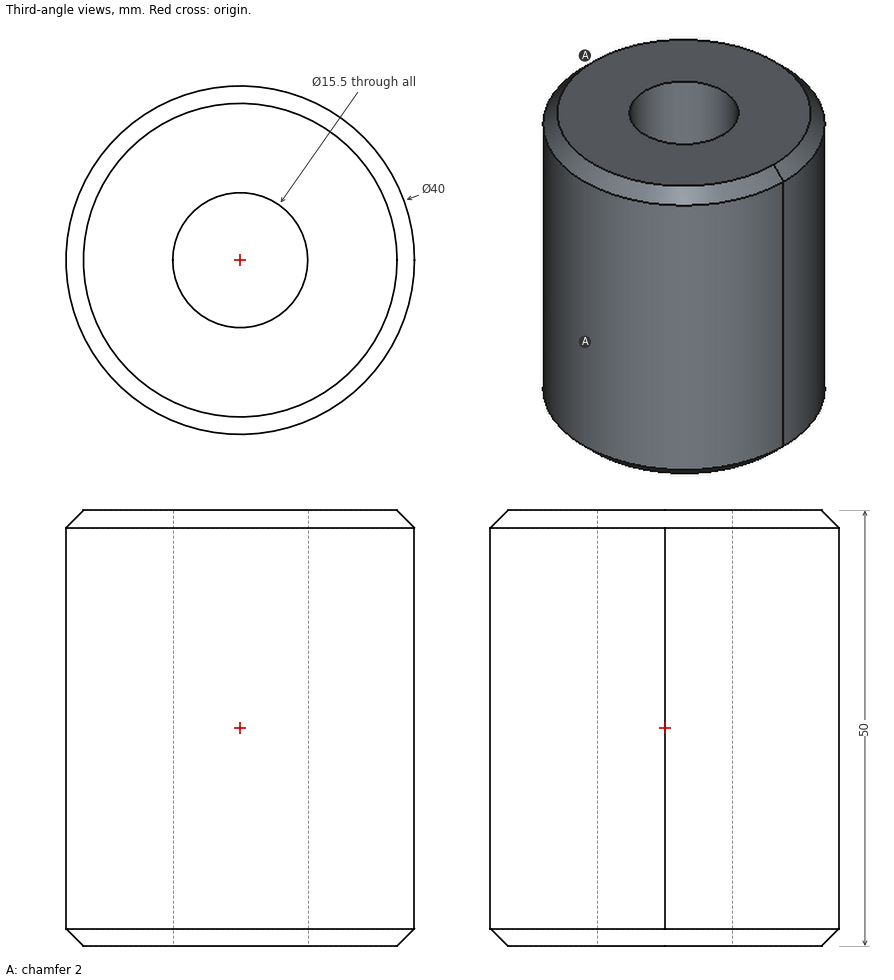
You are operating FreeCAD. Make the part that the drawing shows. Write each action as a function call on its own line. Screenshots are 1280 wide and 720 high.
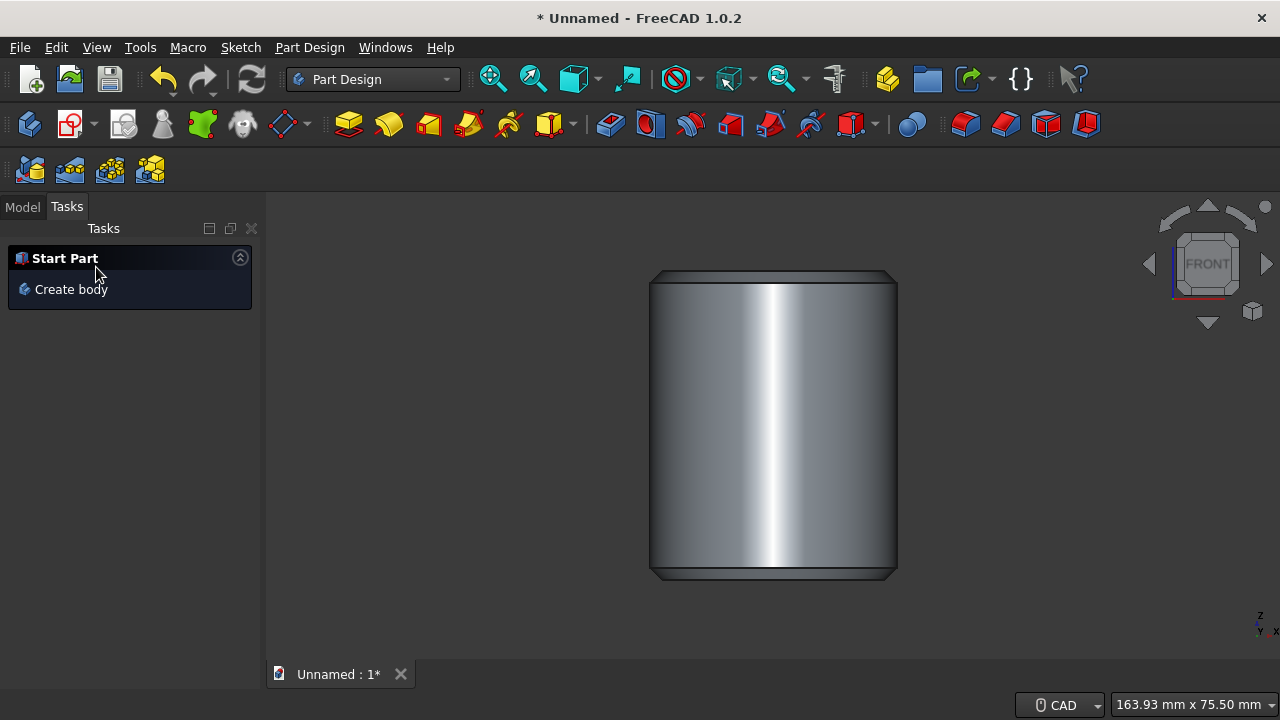
key(0)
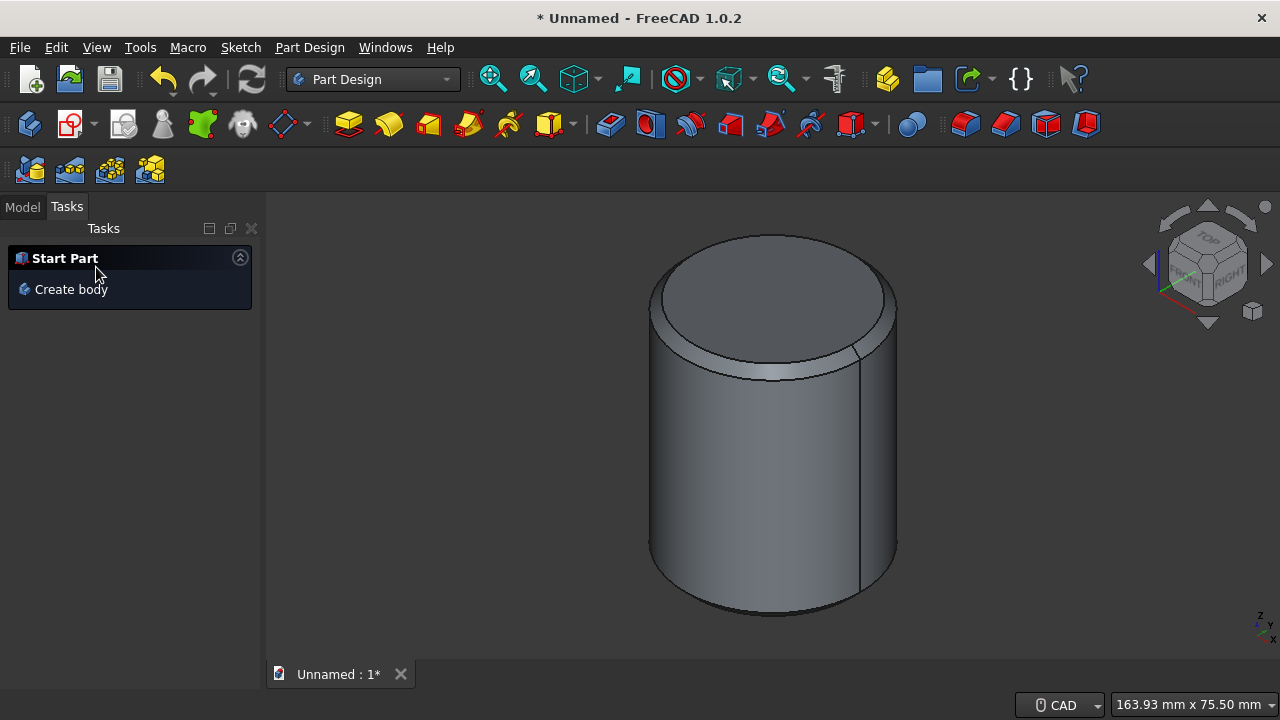
click(773, 298)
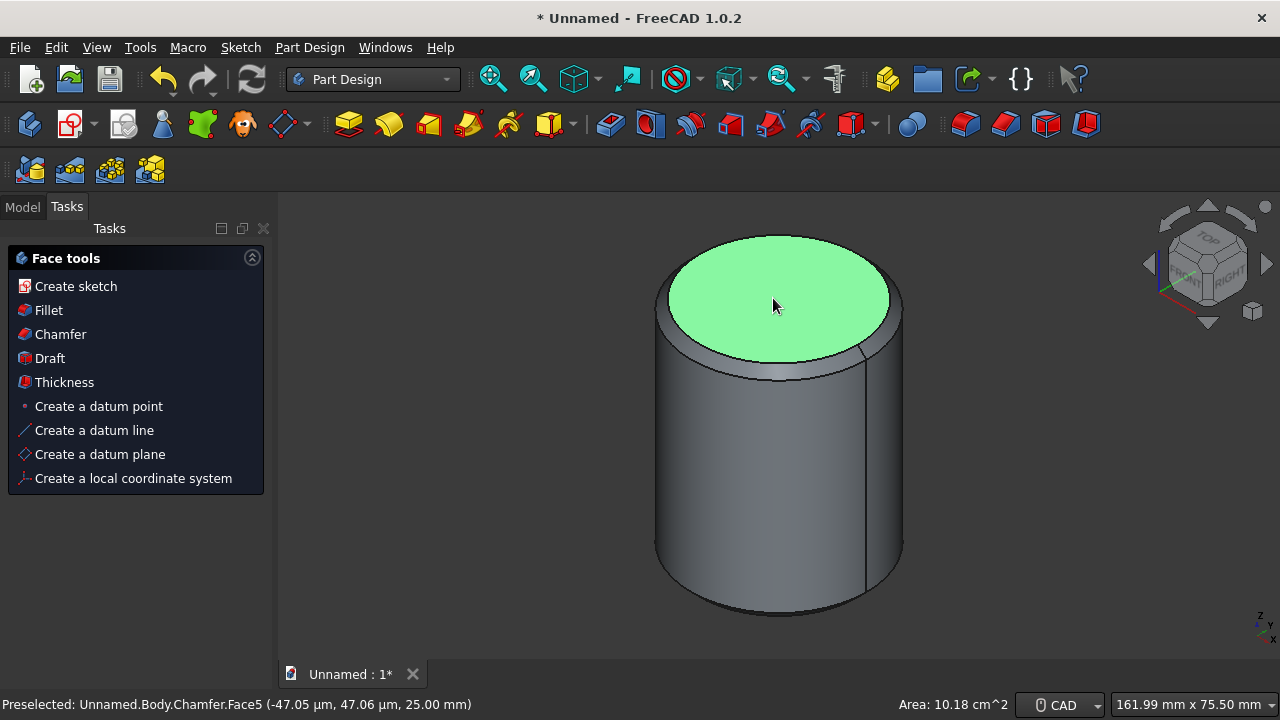
click(70, 124)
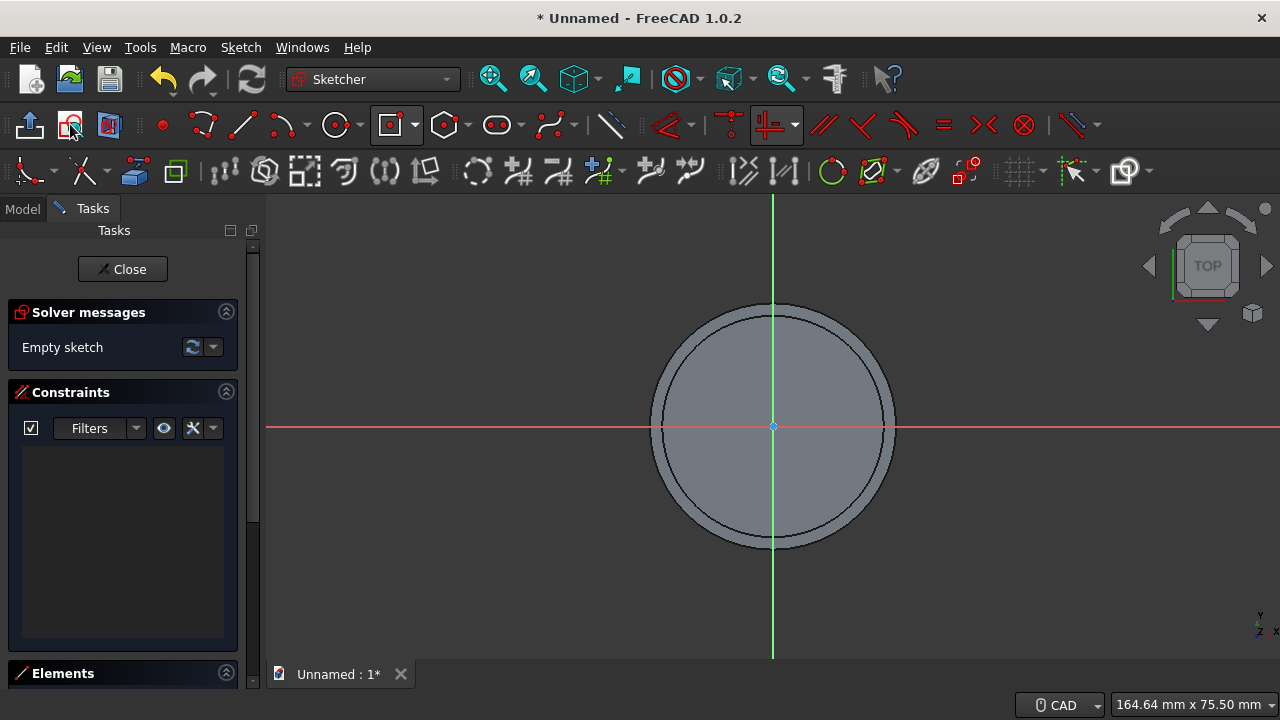
scroll(803, 426, up, 6)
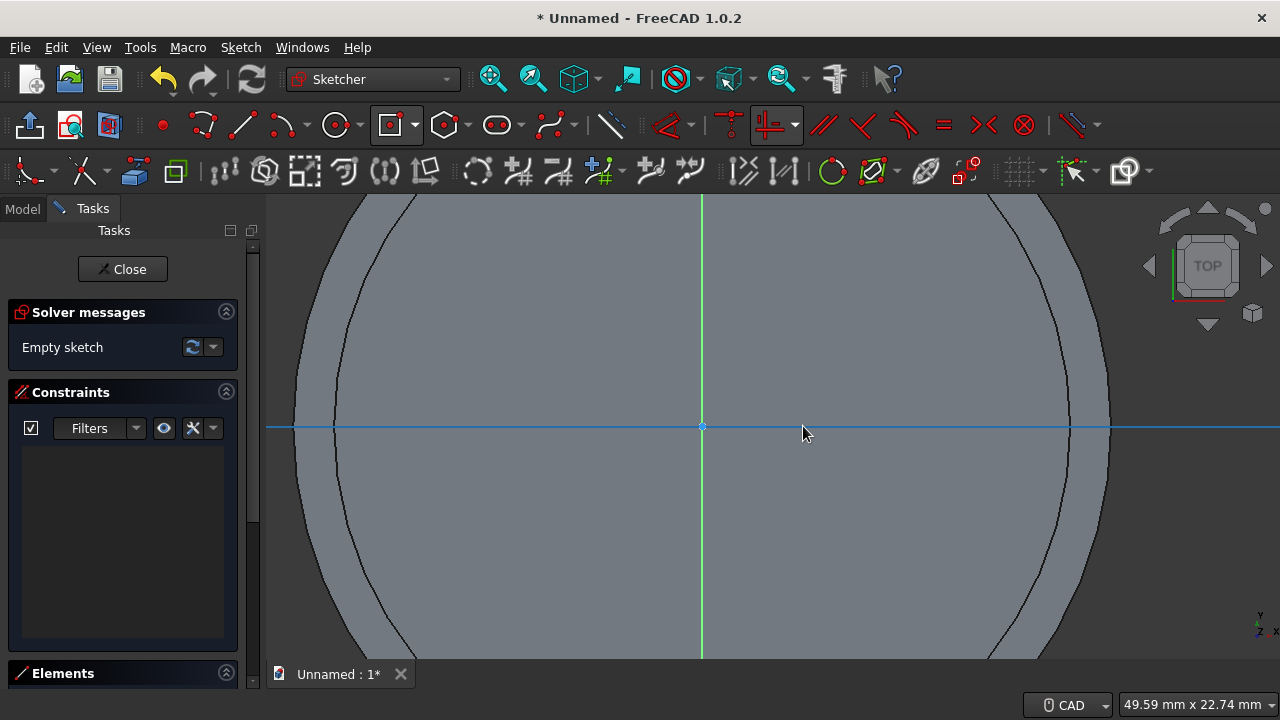
key(g)
key(c)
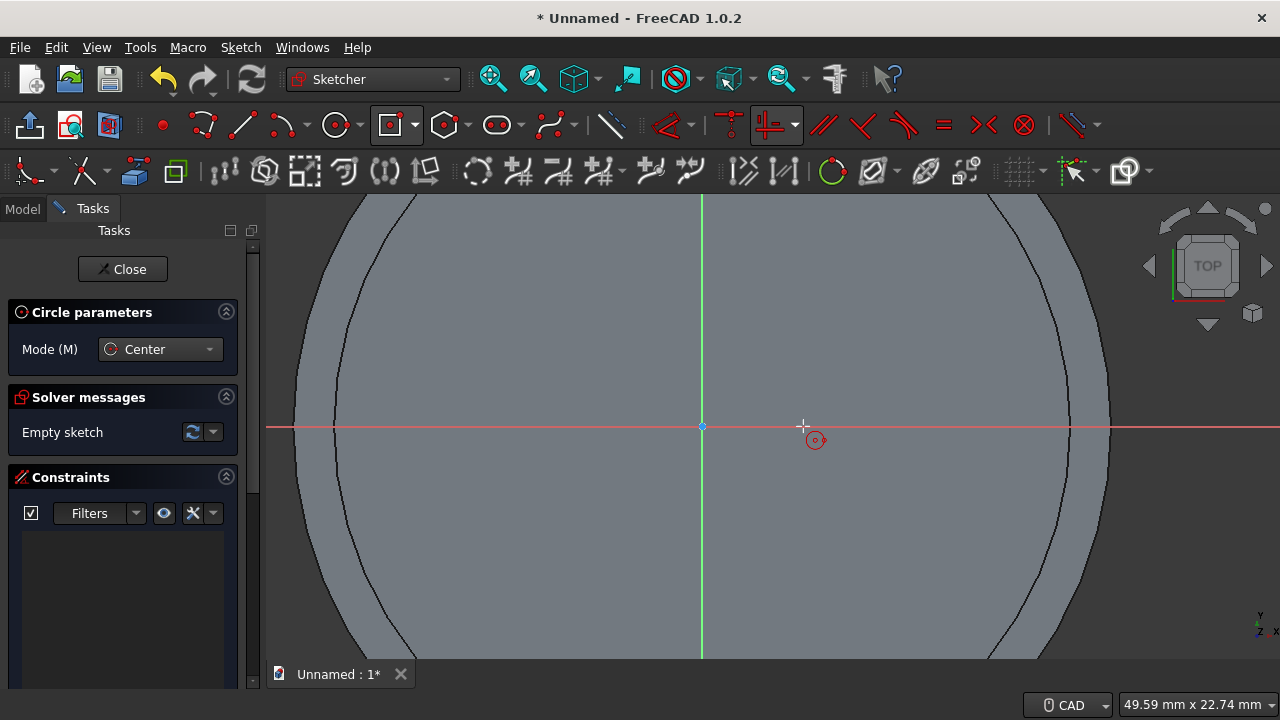
click(702, 426)
move(814, 314)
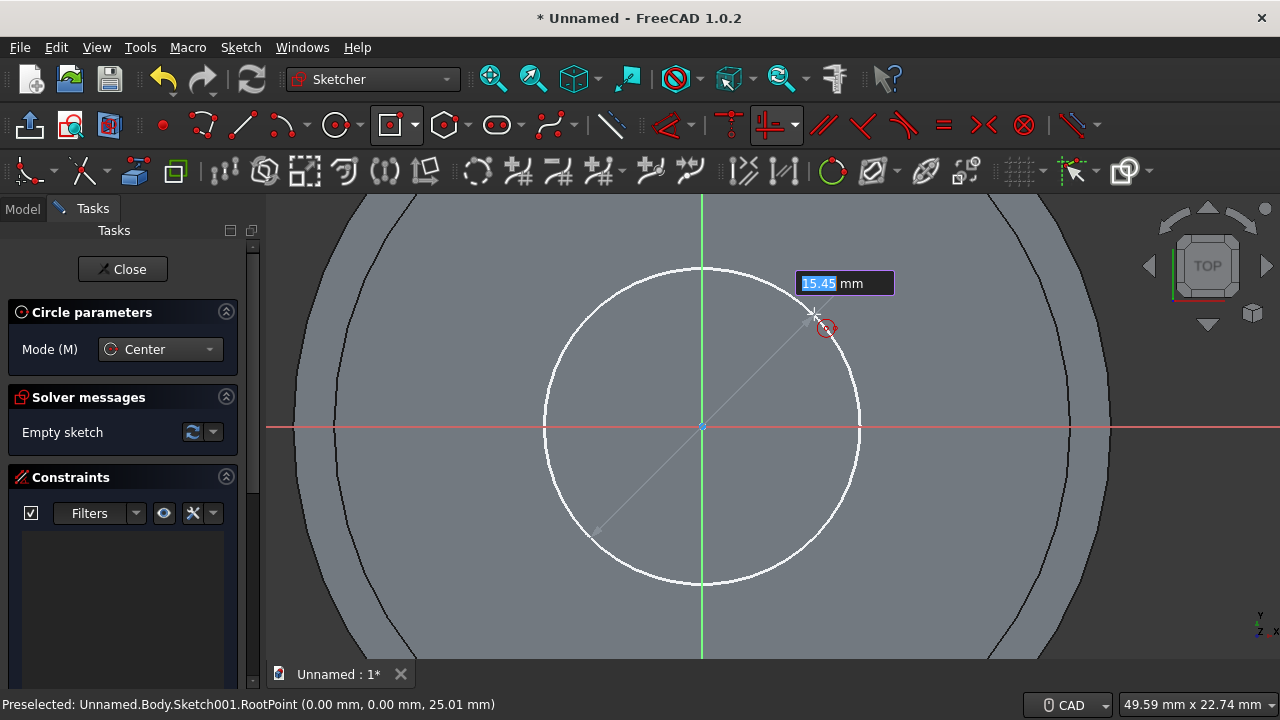
text(15.5)
key(Return)
key(Escape)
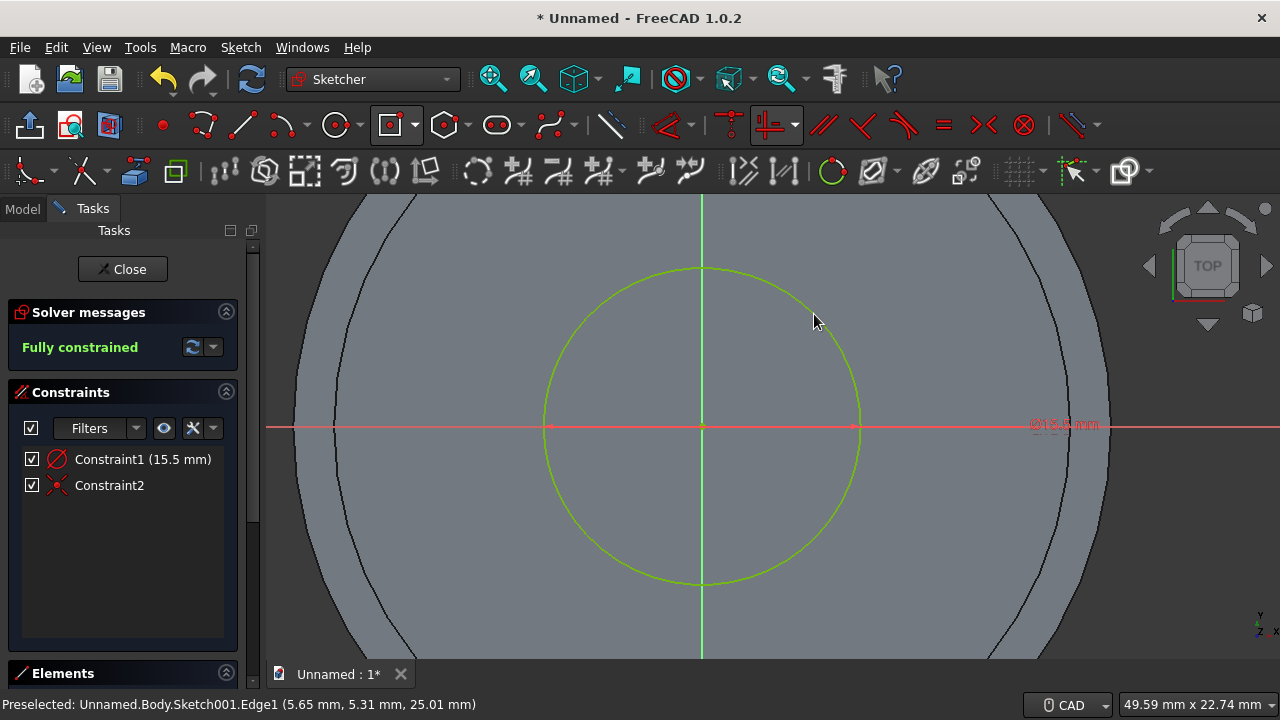
click(123, 269)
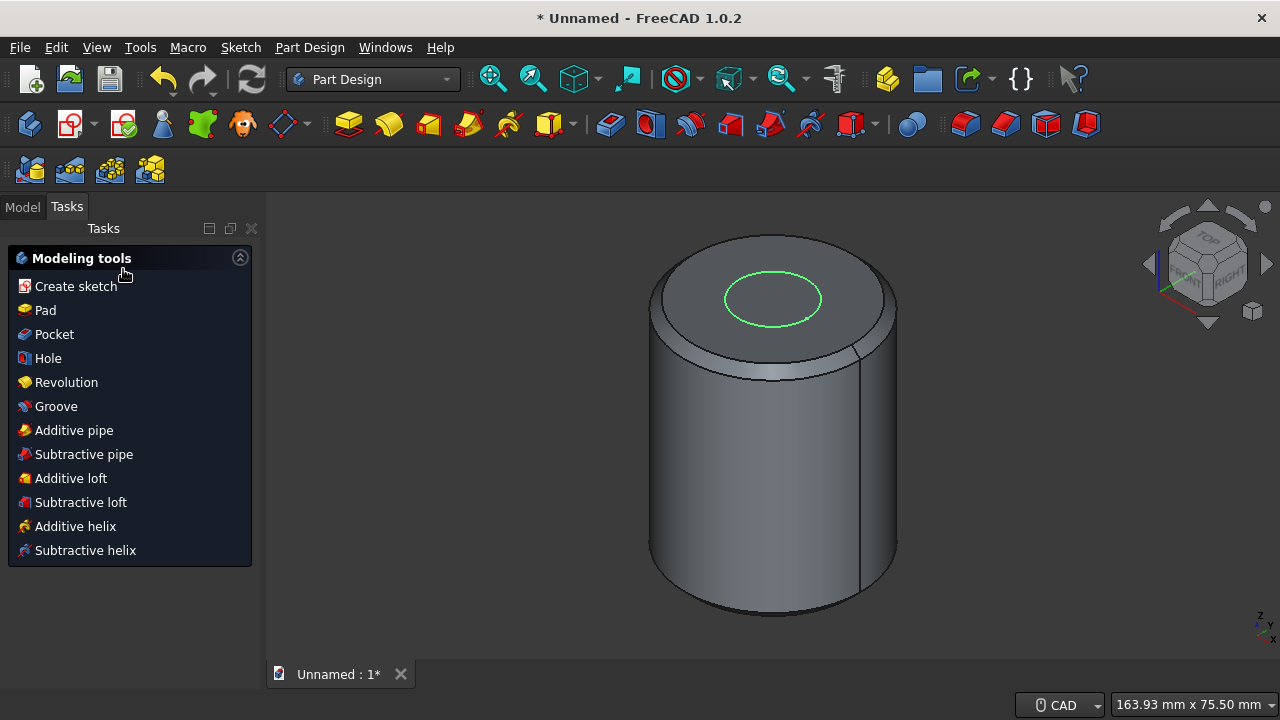
click(652, 124)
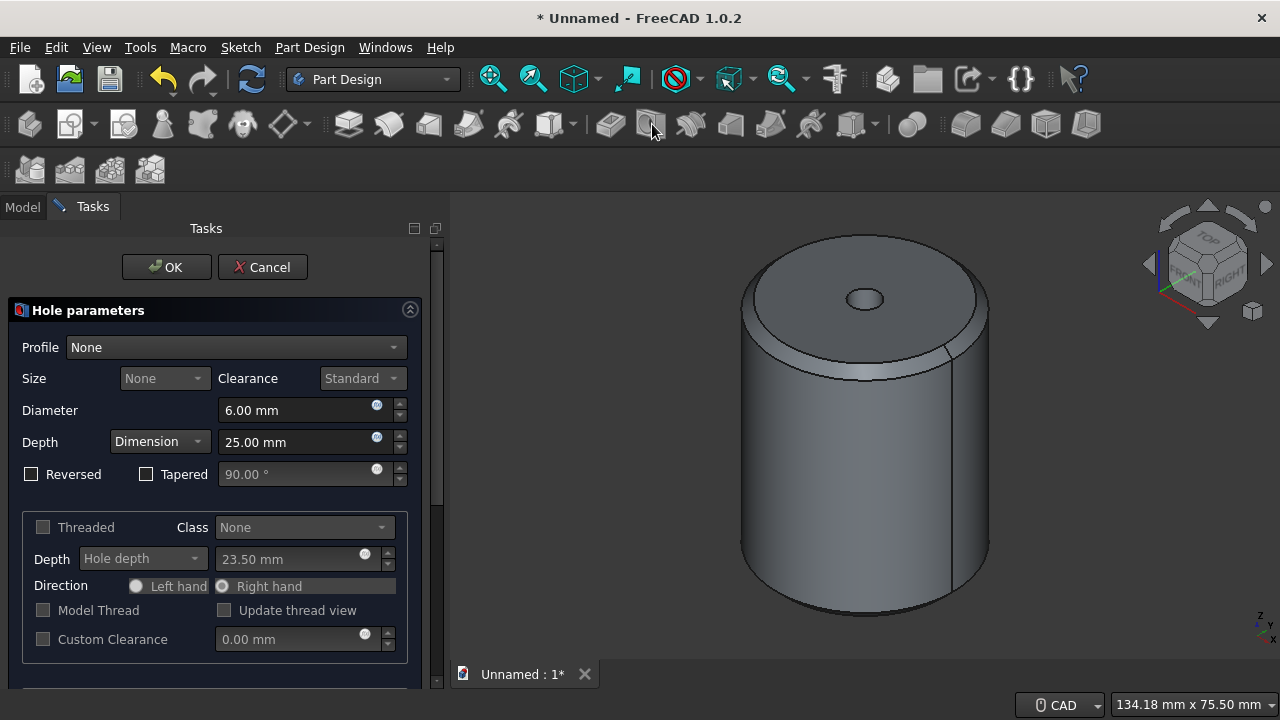
triple_click(305, 410)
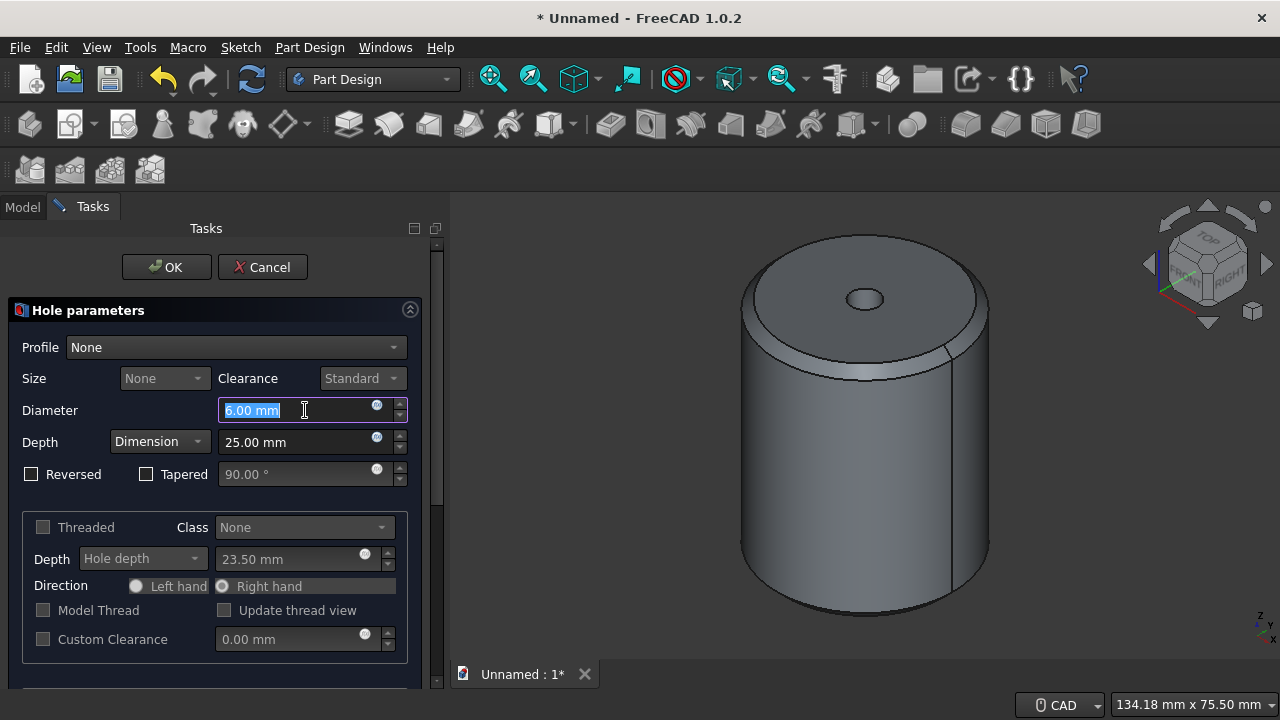
text(15.5)
key(Tab)